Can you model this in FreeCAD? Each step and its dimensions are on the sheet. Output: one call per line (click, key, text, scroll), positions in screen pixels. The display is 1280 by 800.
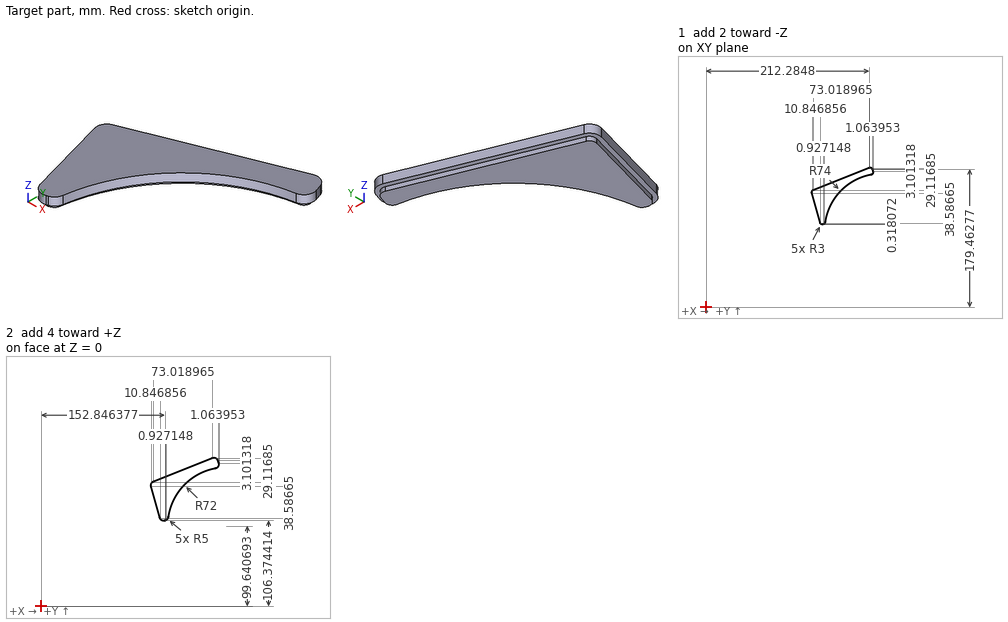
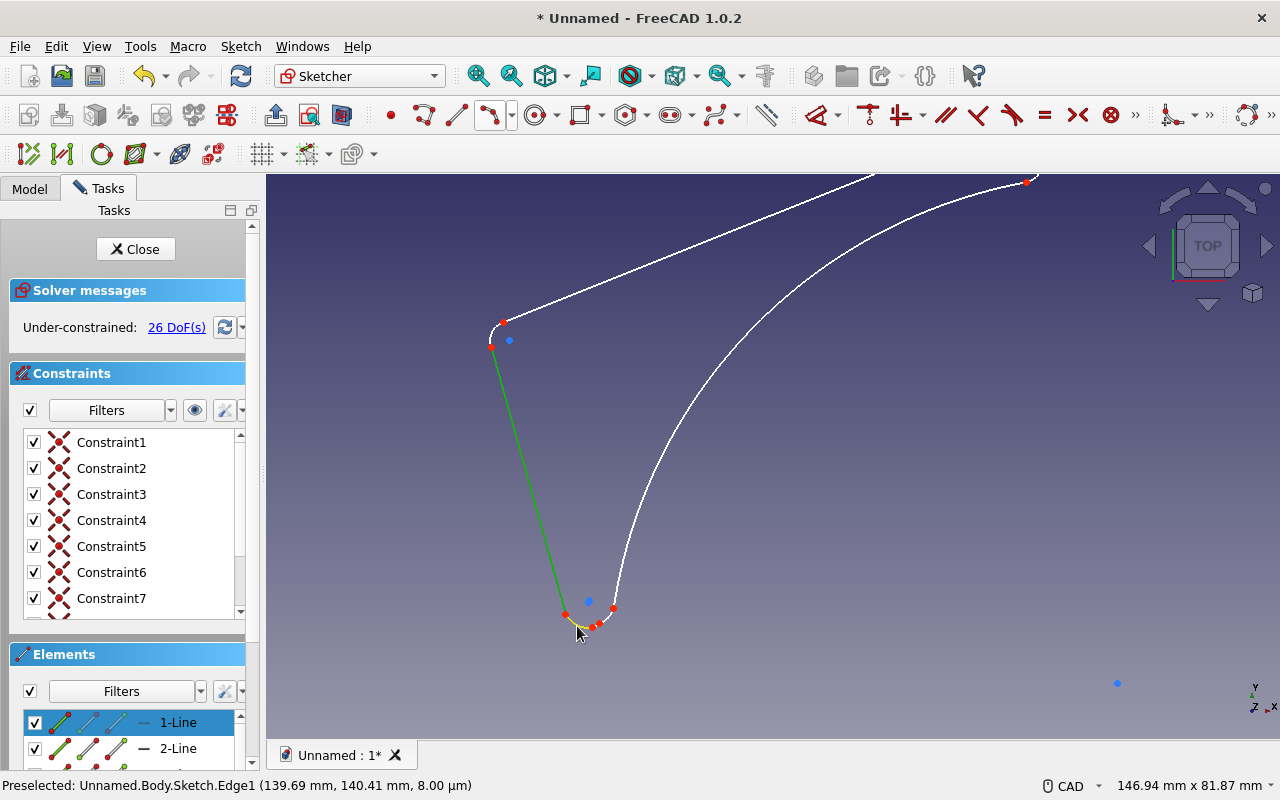
click(577, 625)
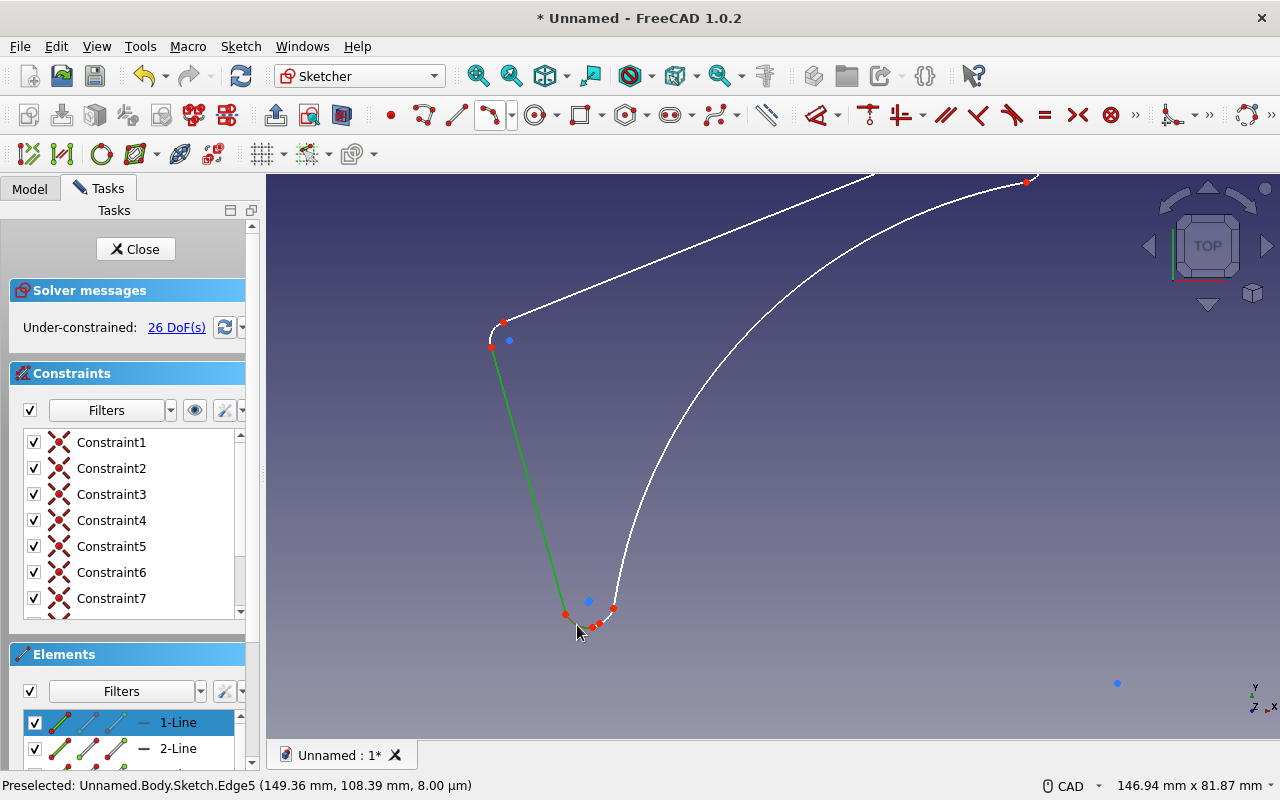
click(1012, 116)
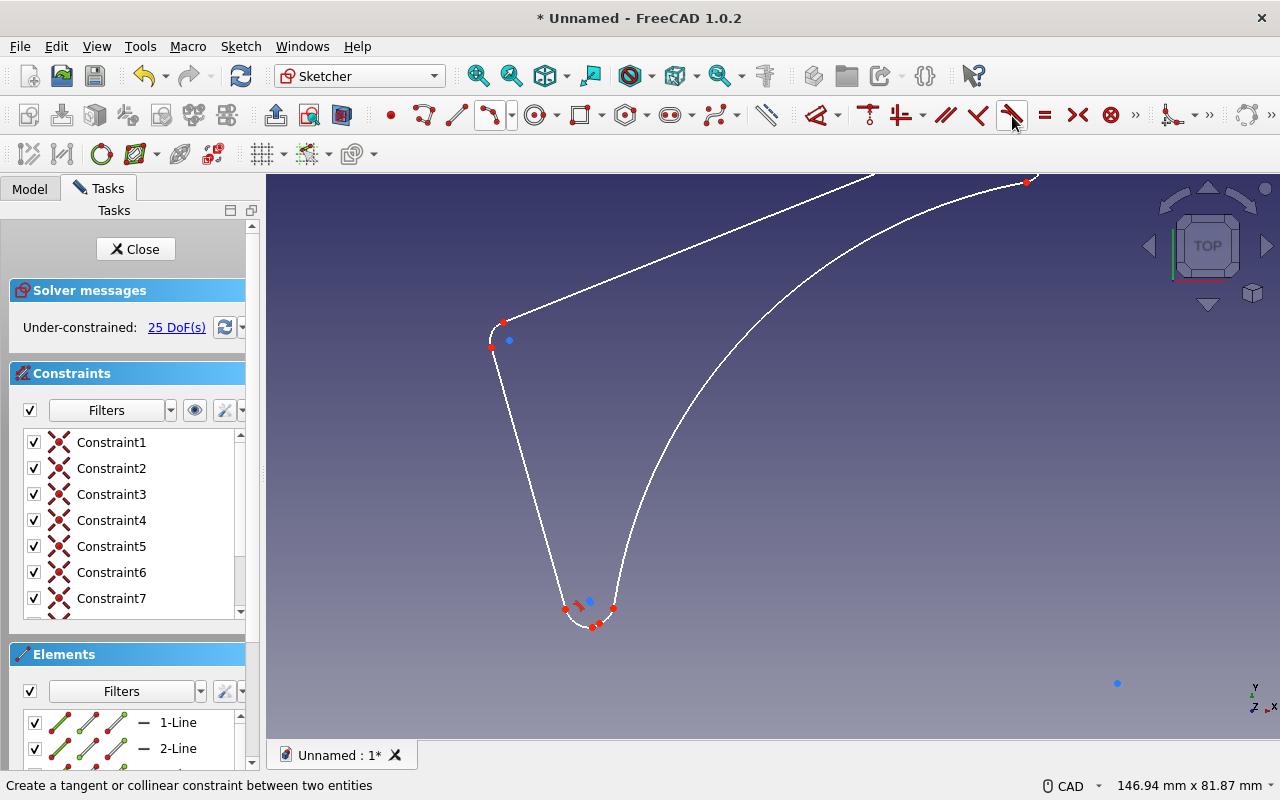
click(514, 426)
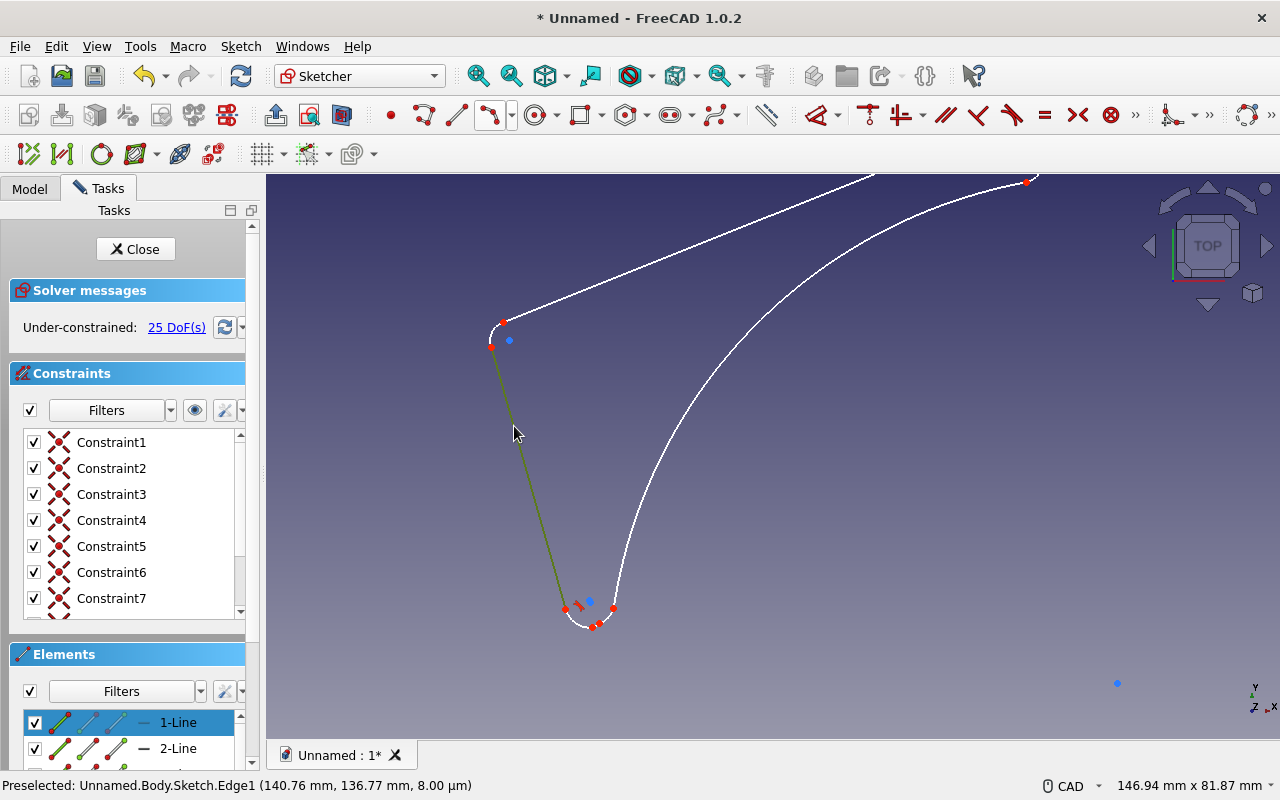
scroll(496, 327, up, 3)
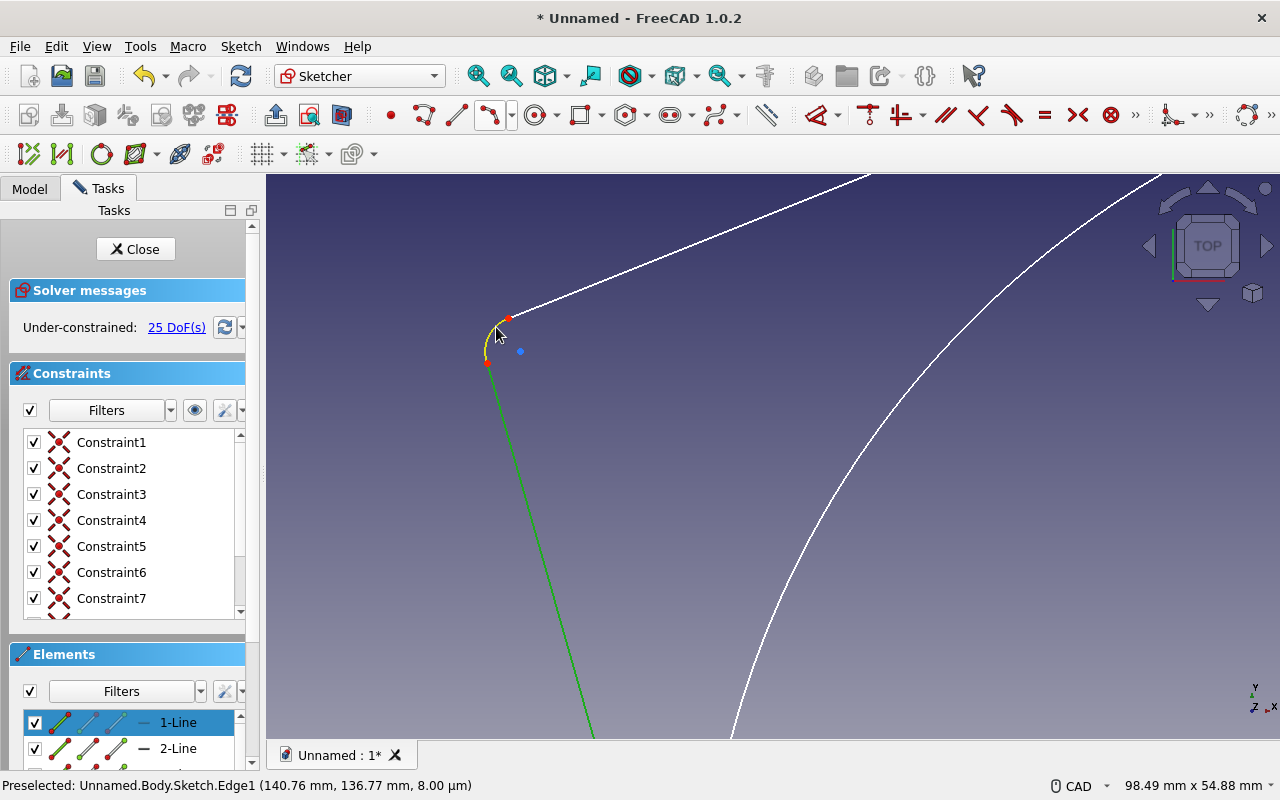
click(495, 327)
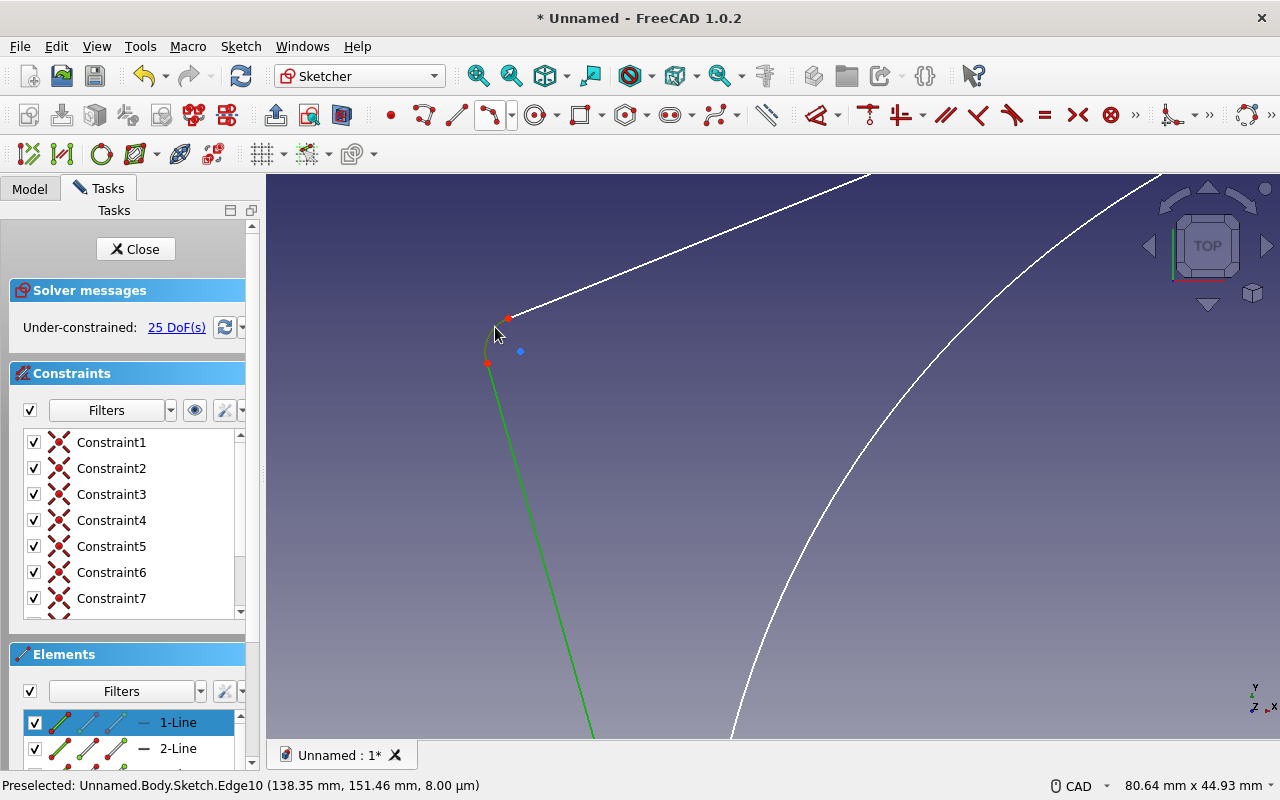
click(1012, 116)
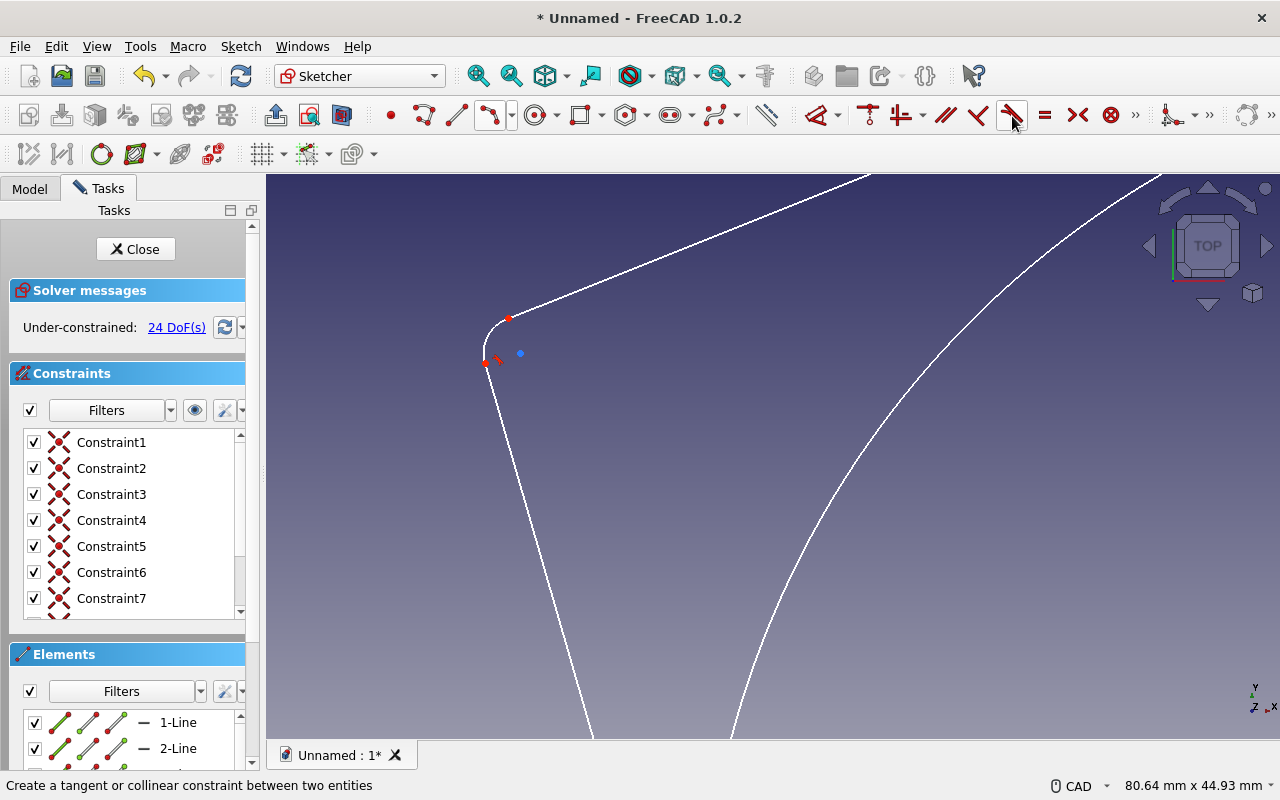
scroll(539, 483, down, 5)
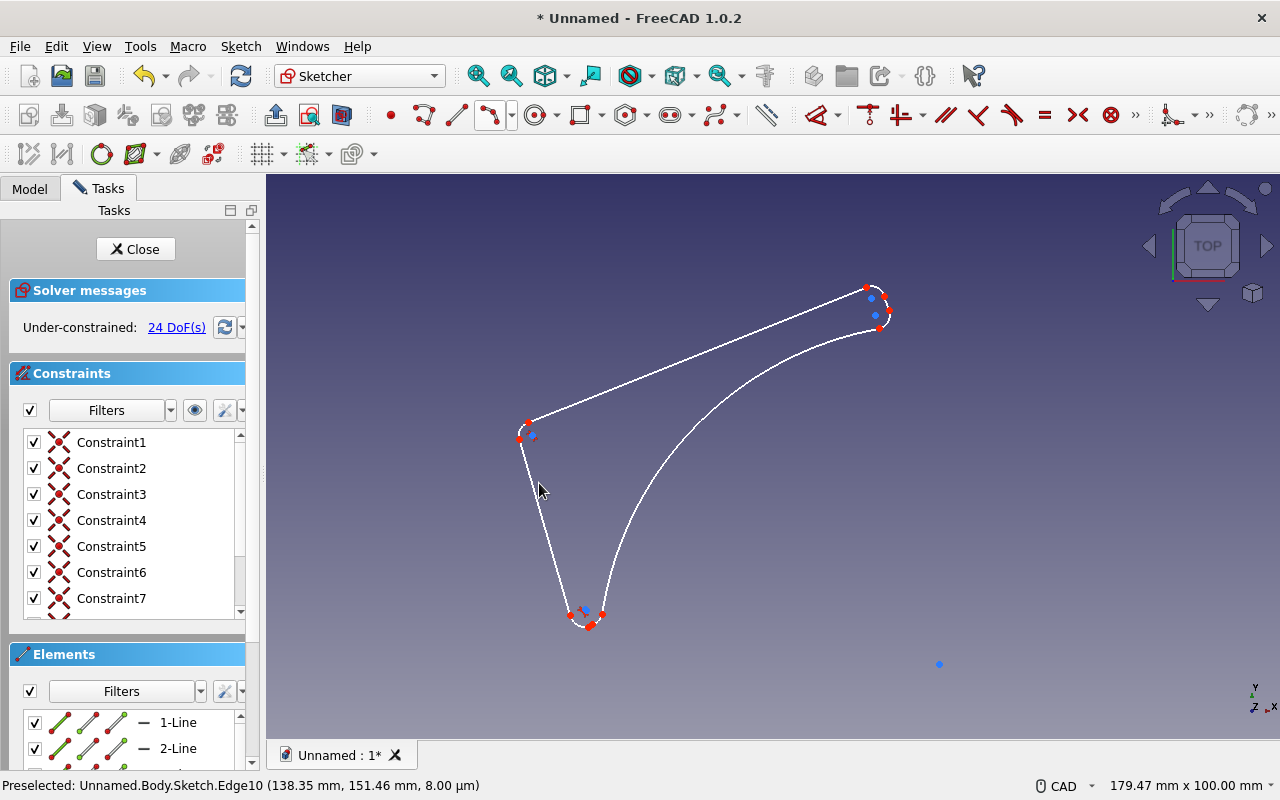
scroll(590, 626, up, 9)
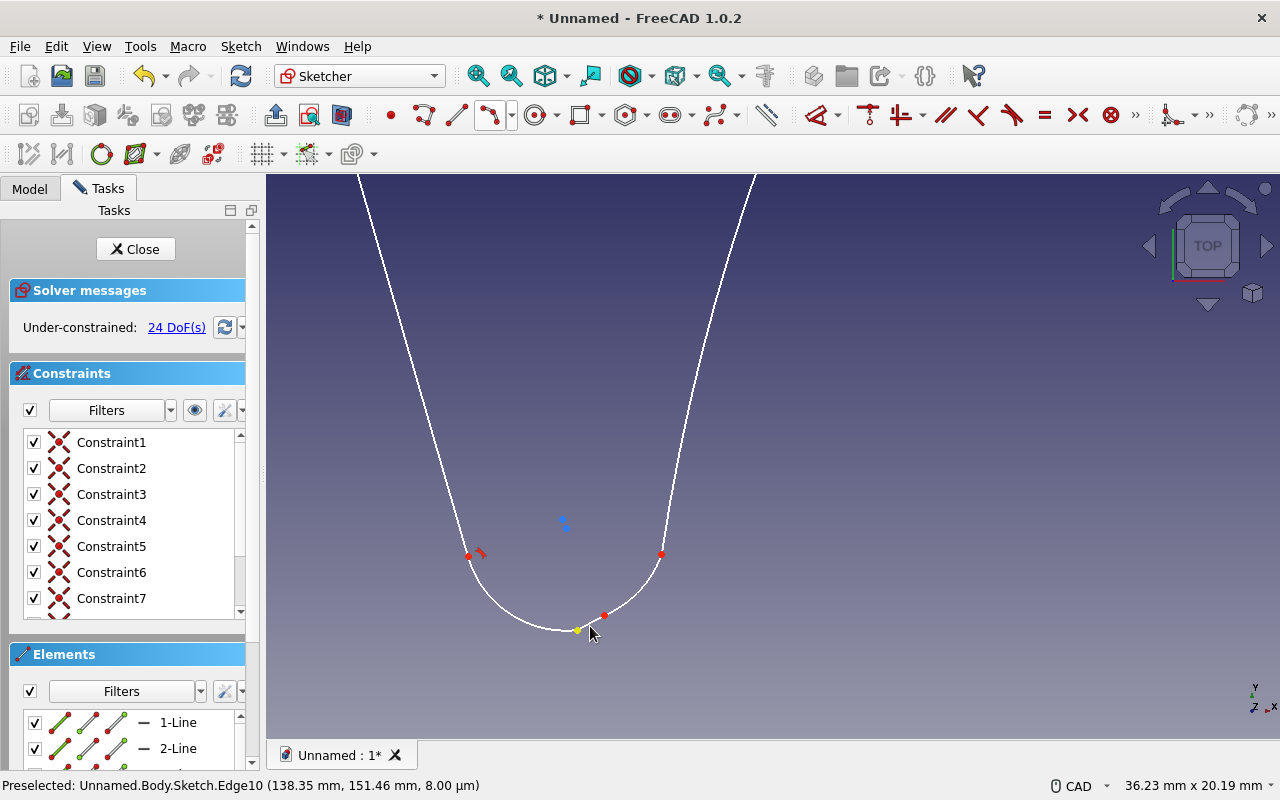
click(591, 623)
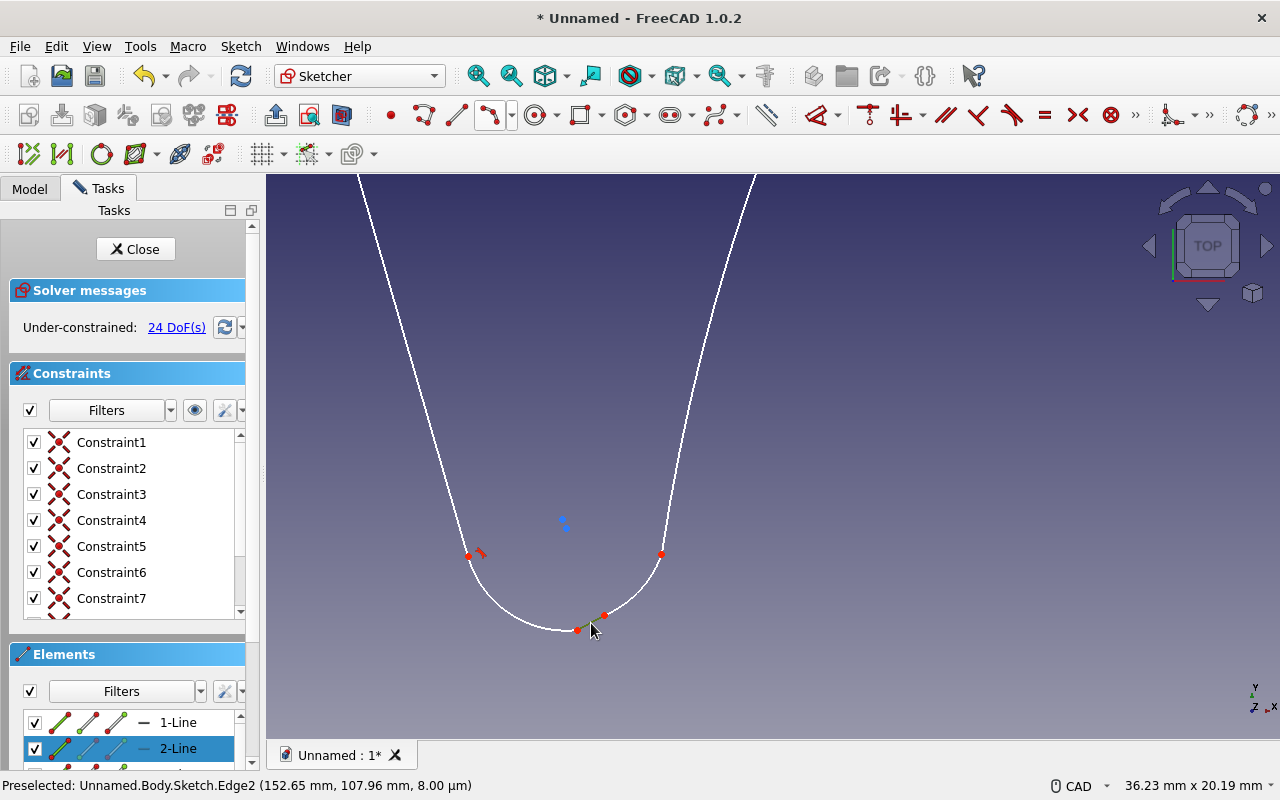
scroll(590, 627, down, 9)